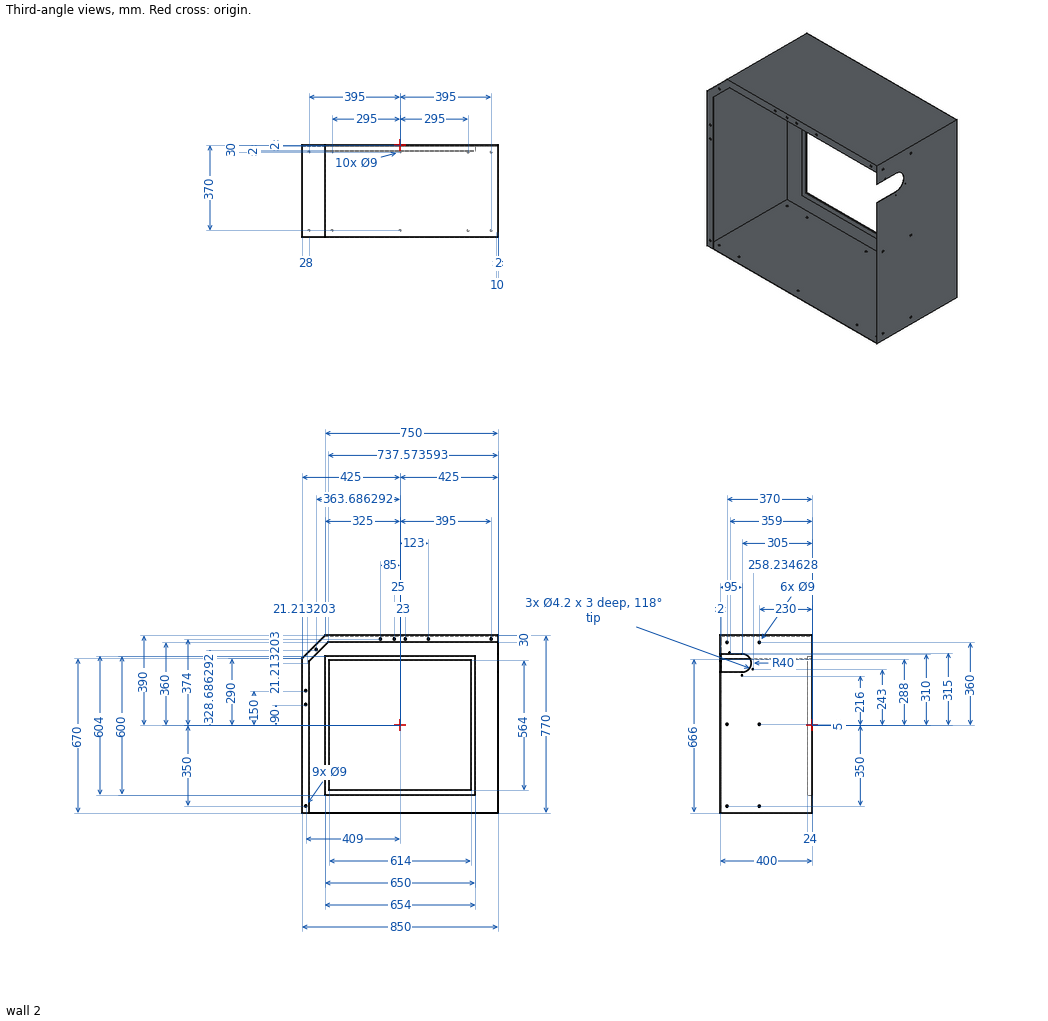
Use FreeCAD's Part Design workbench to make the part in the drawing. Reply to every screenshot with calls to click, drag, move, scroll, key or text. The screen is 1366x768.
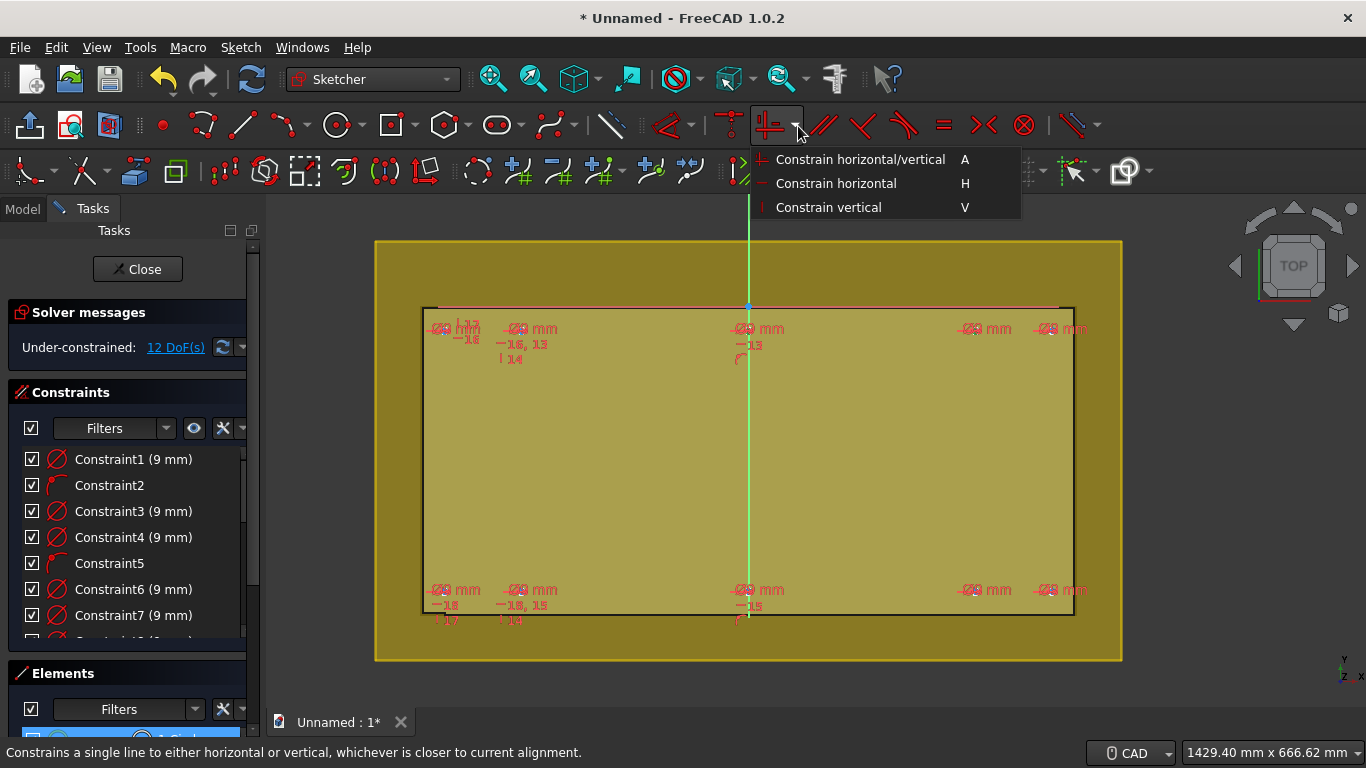
click(886, 183)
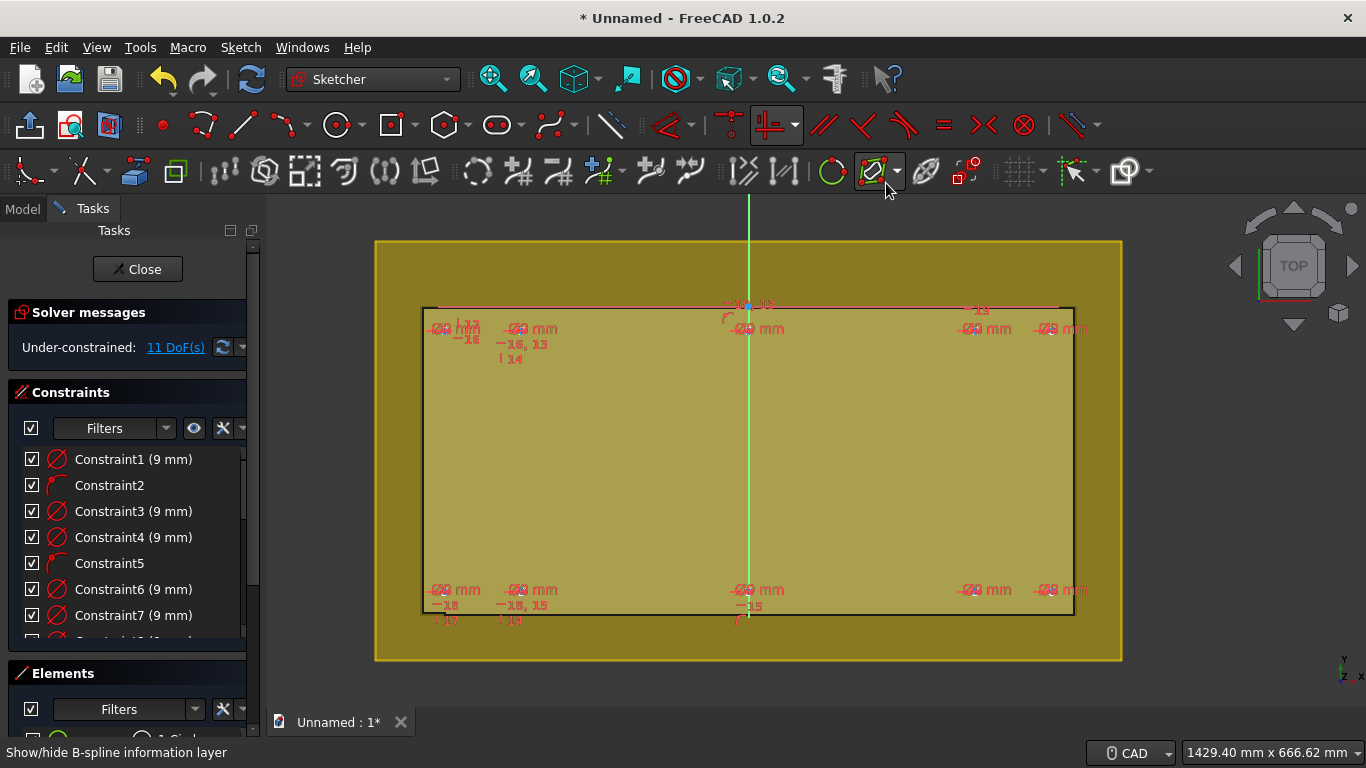
click(976, 331)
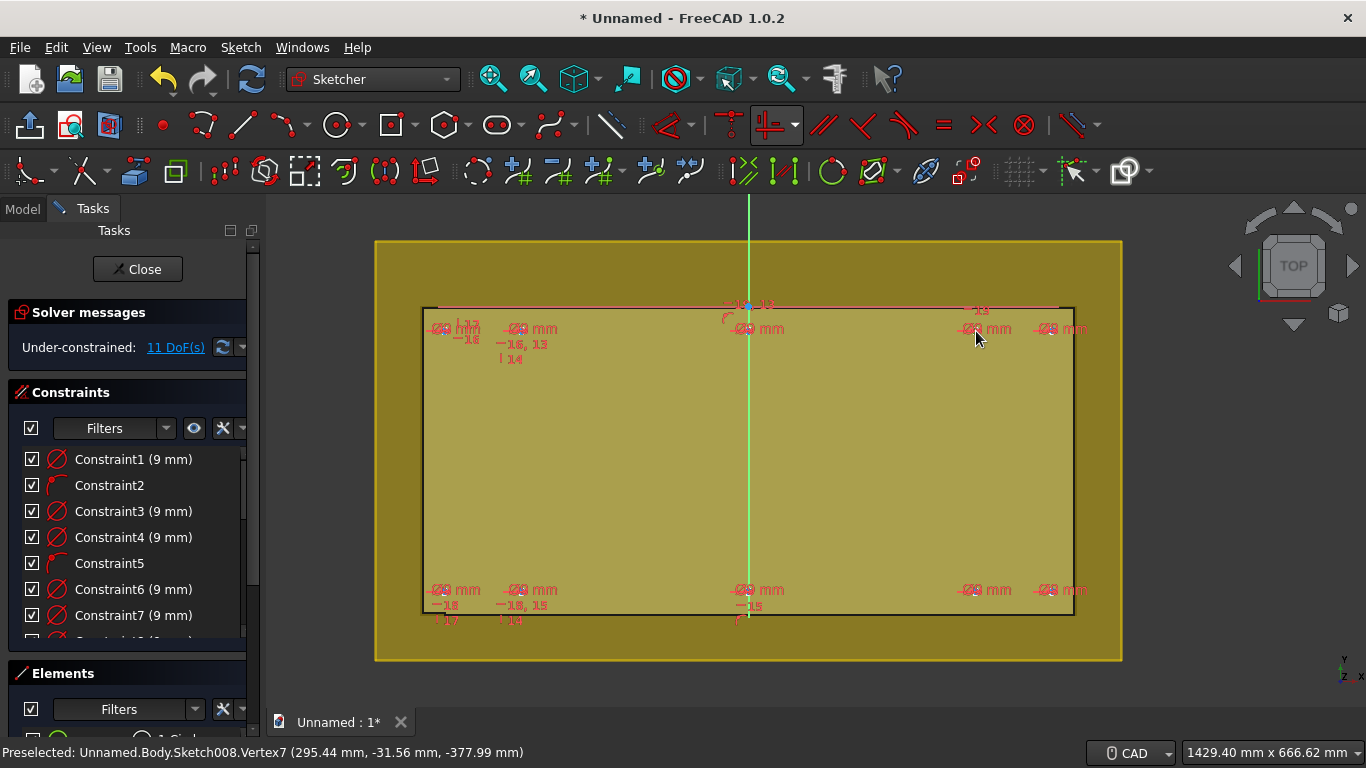
click(976, 592)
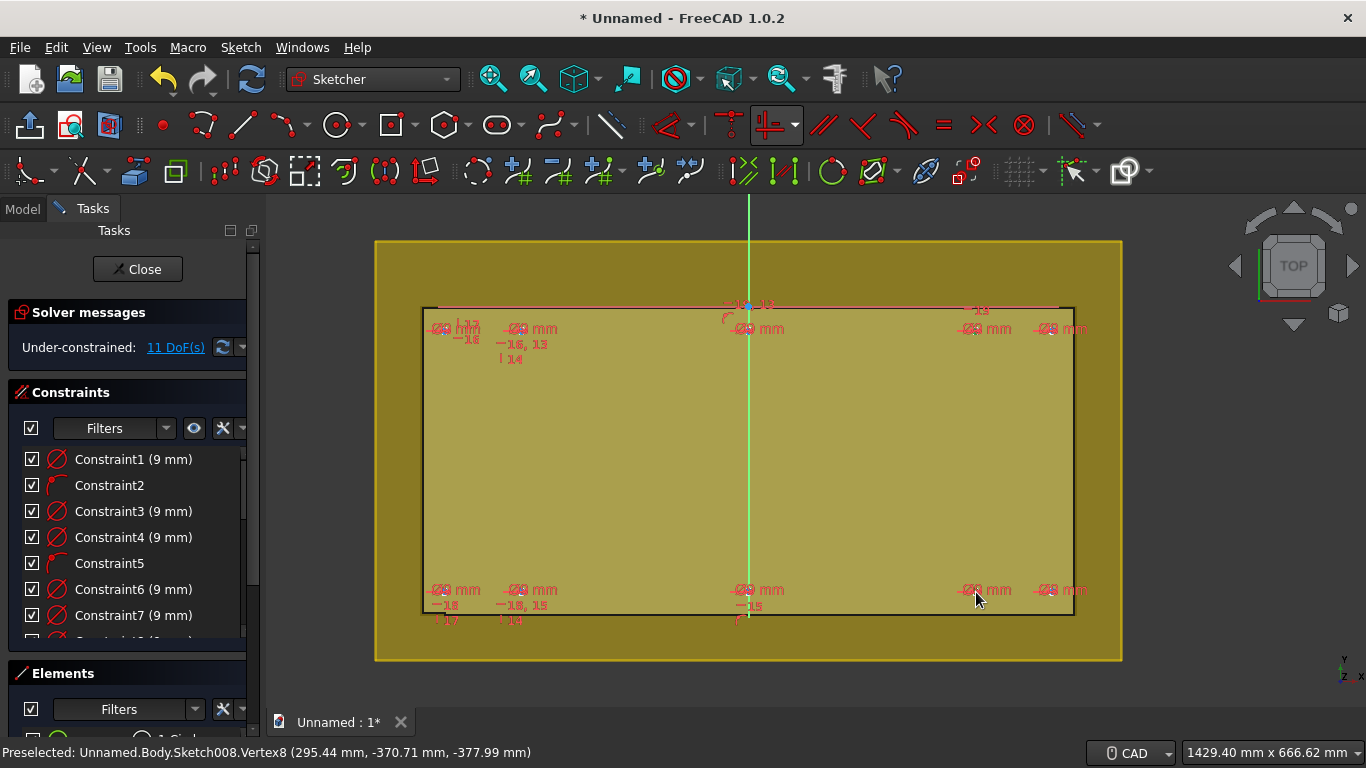
click(798, 126)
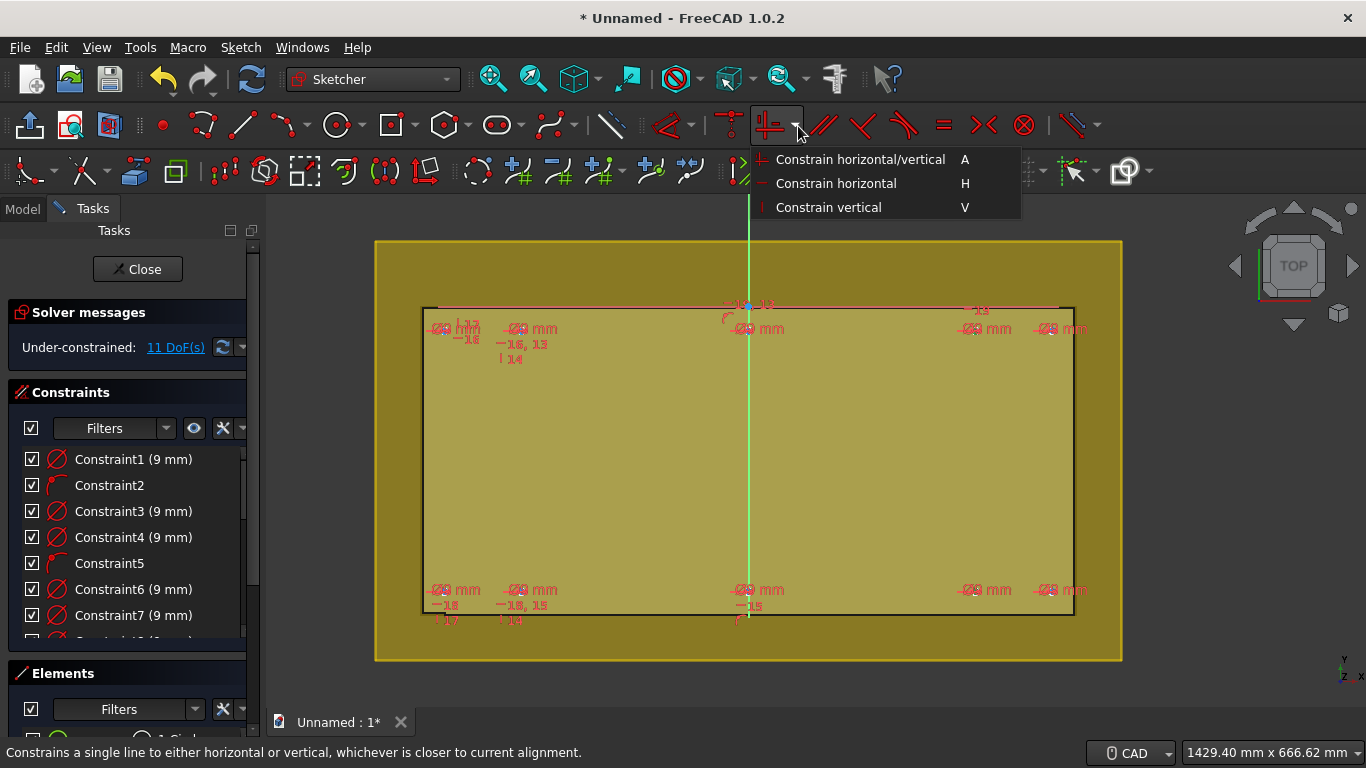
click(886, 207)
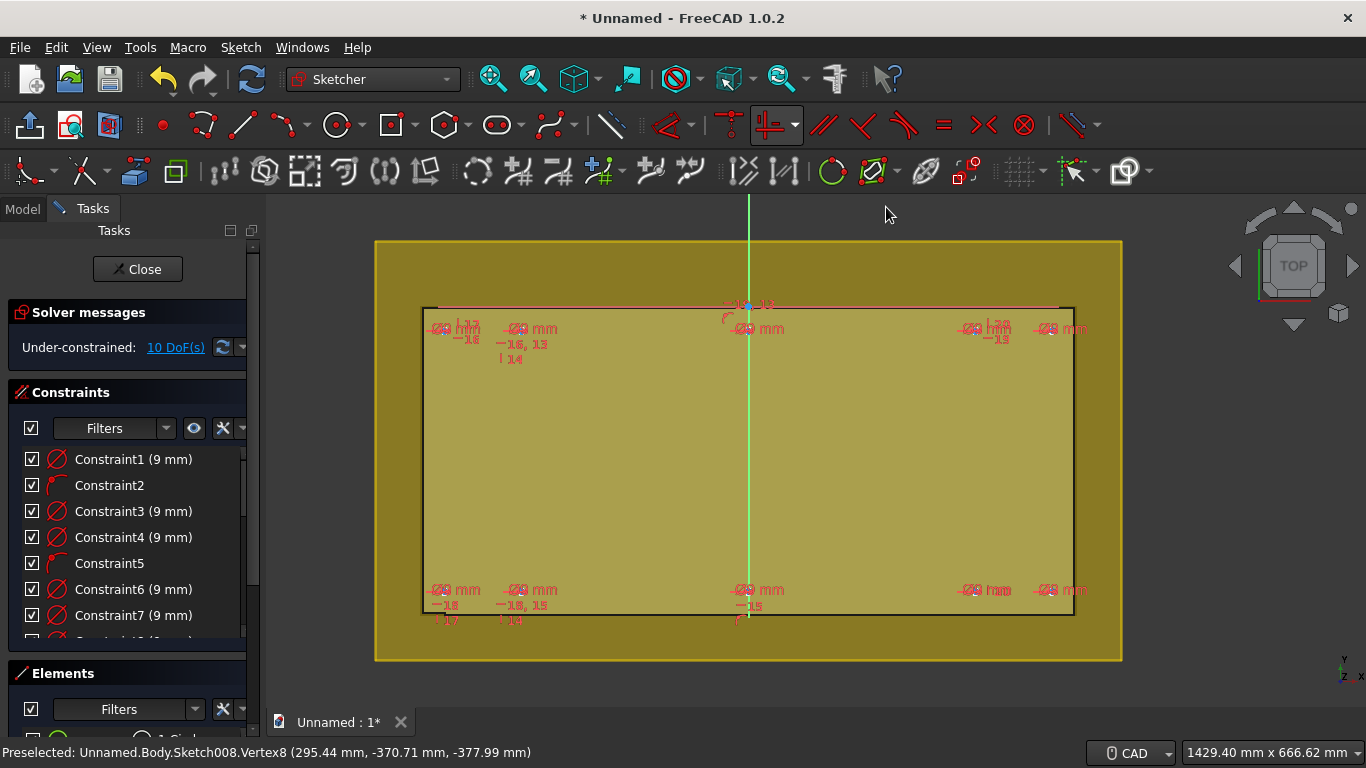
click(749, 592)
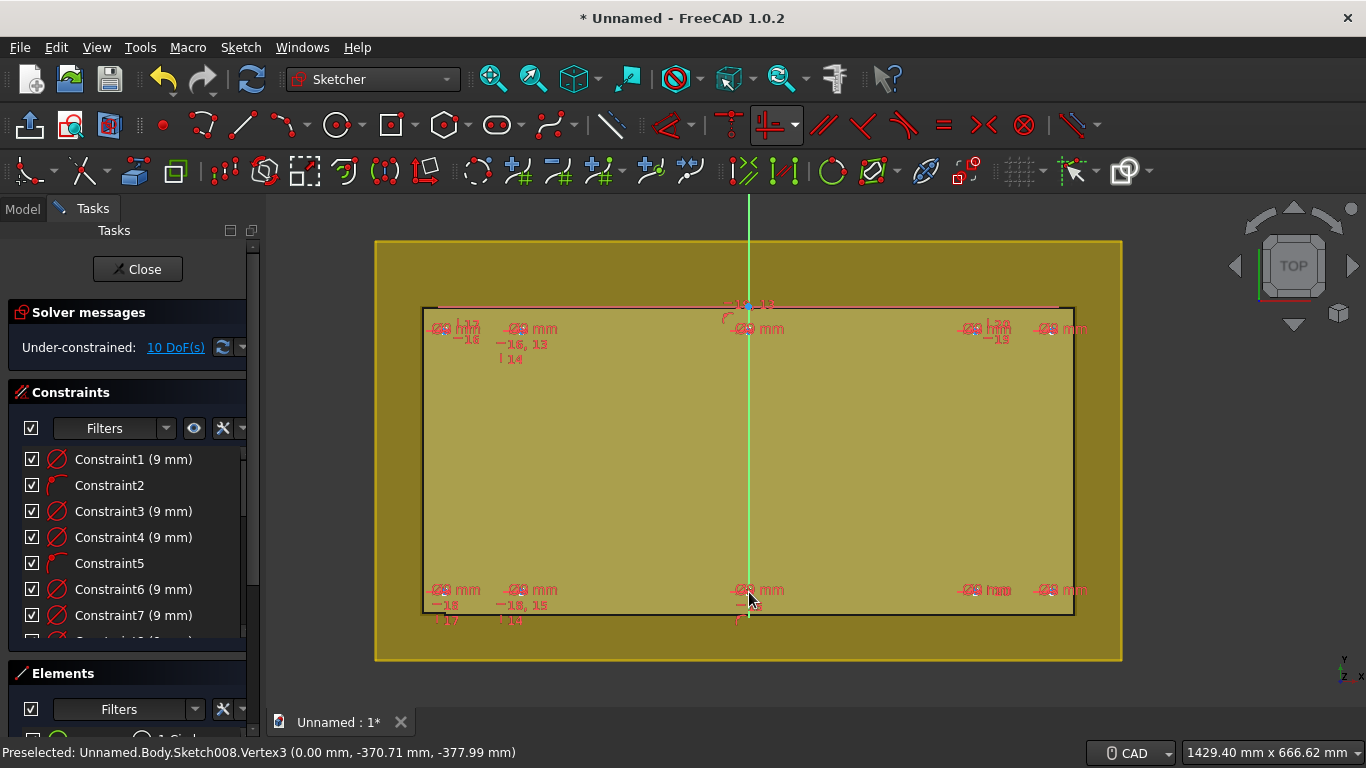
click(976, 592)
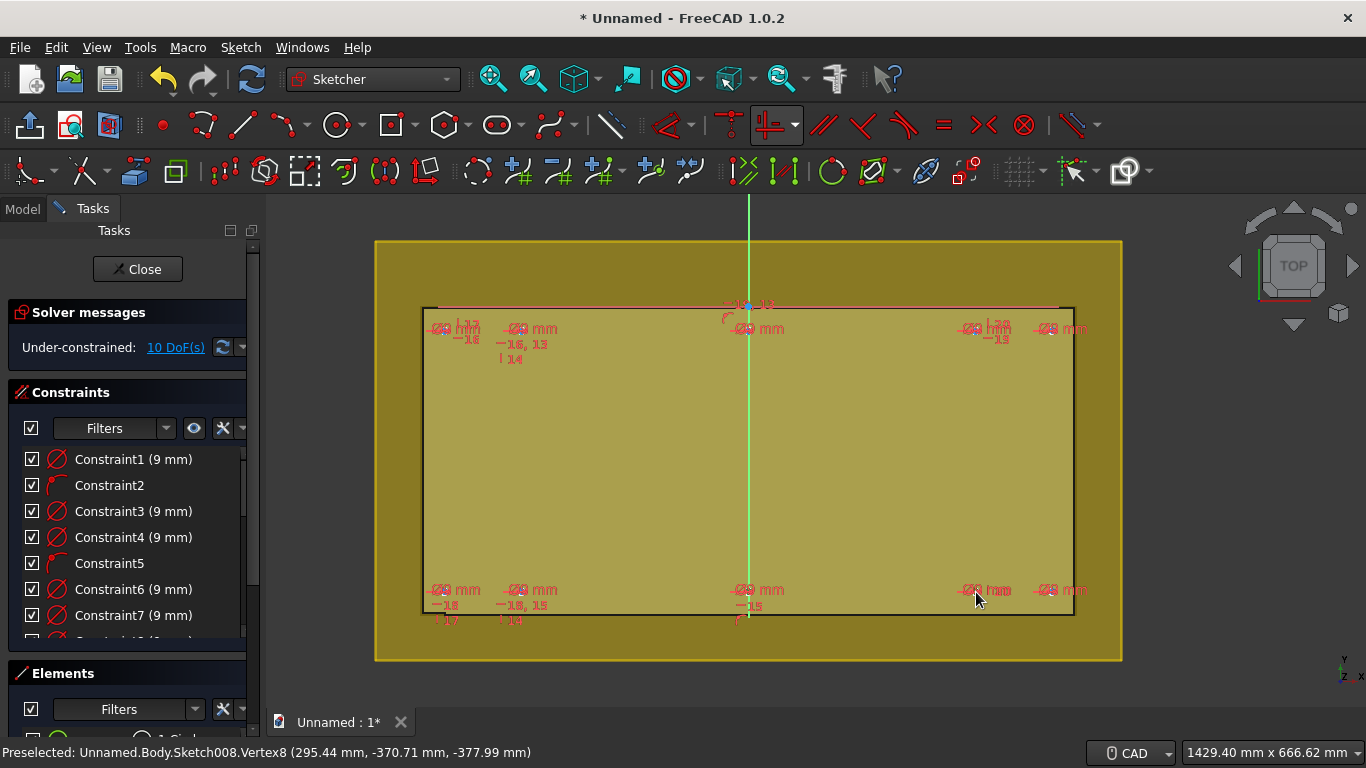
click(798, 126)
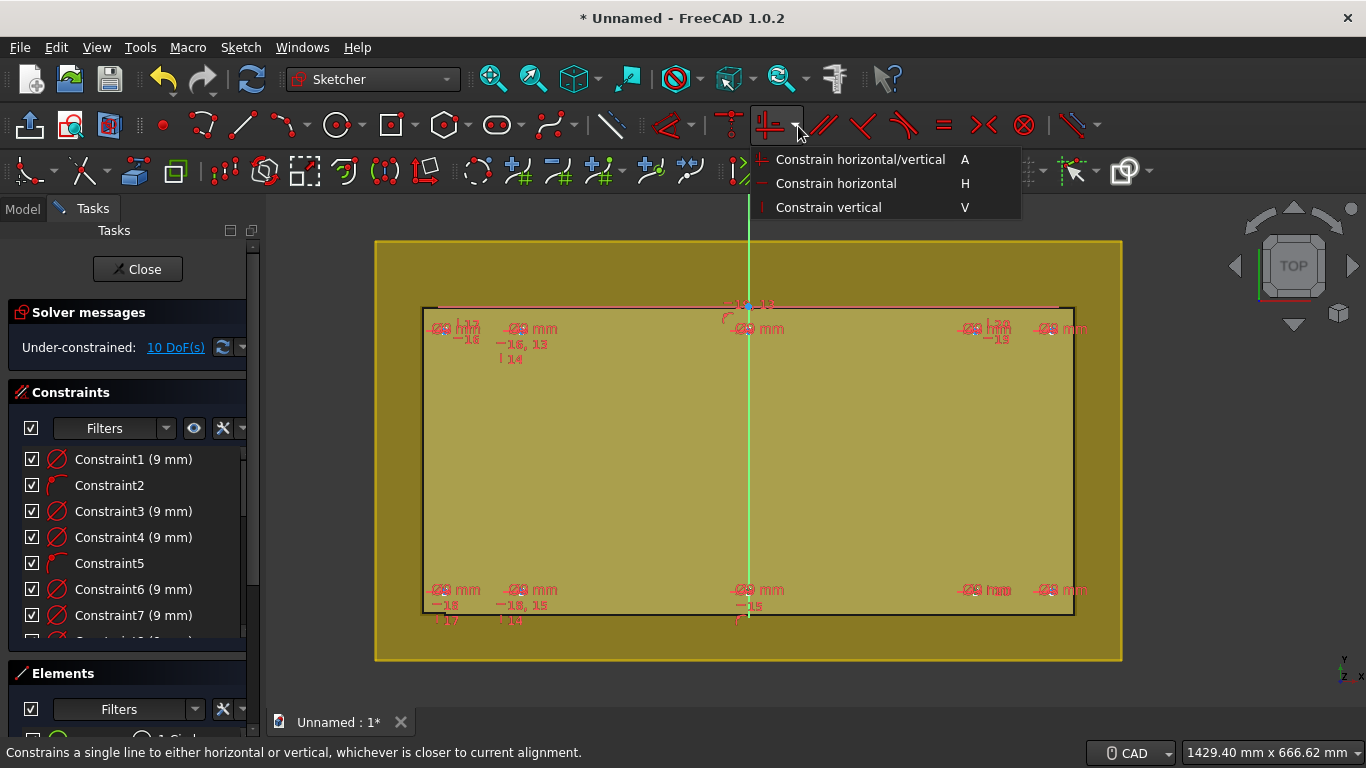
click(886, 183)